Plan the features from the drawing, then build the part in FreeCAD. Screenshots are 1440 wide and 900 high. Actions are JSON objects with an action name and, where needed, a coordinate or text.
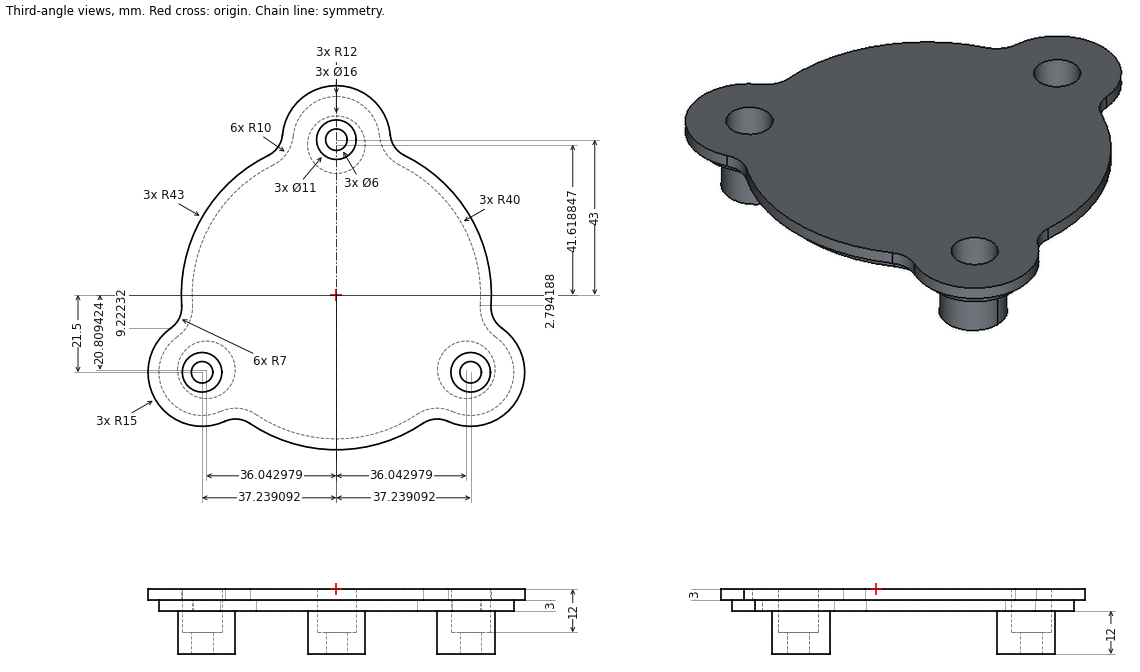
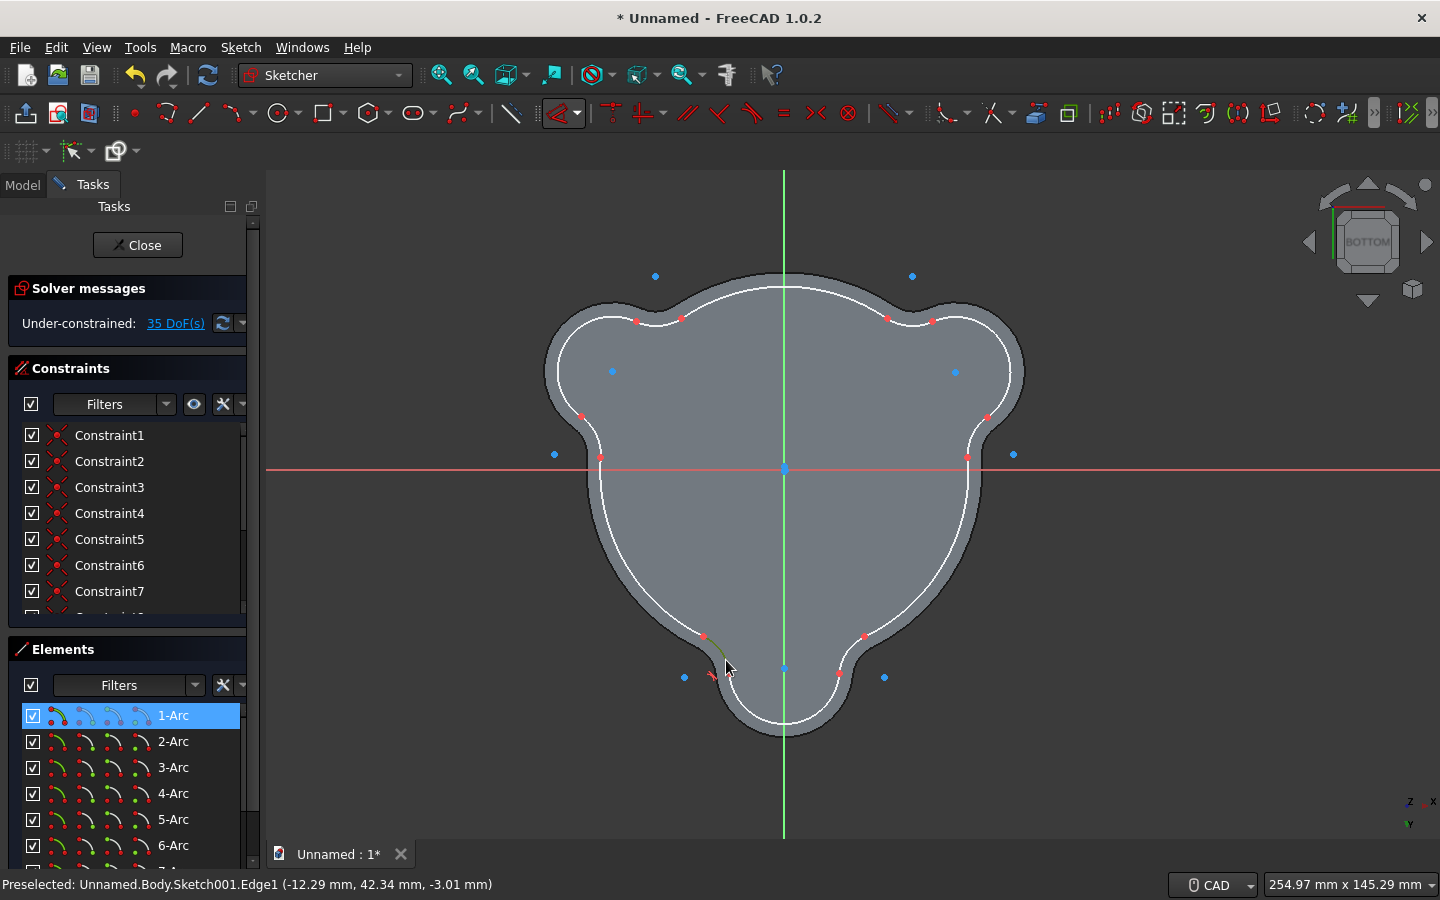
{"action": "left_click", "coordinate": [608, 523]}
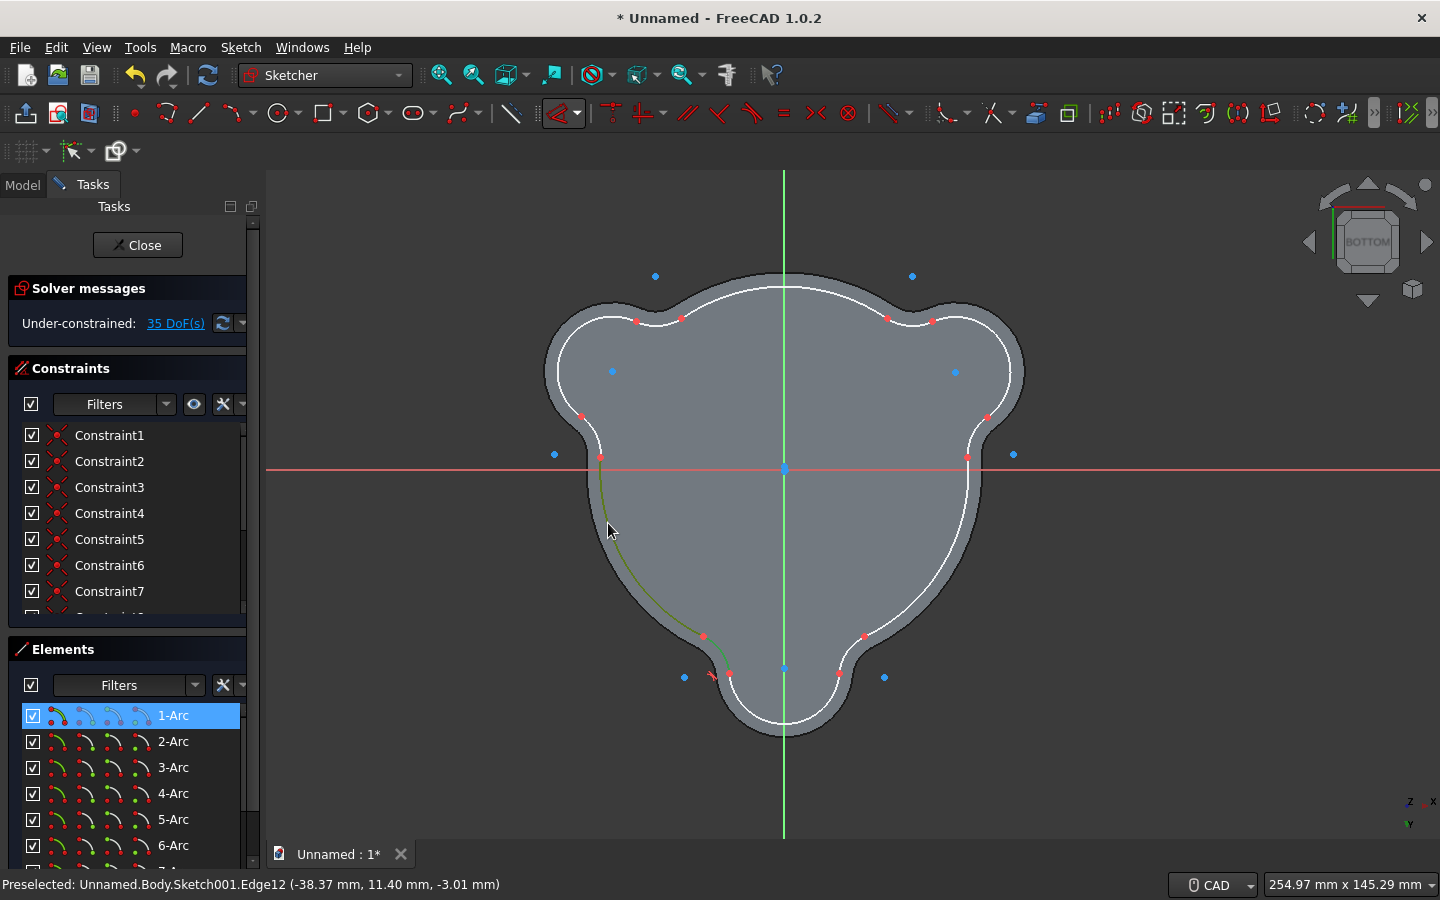
{"action": "left_click", "coordinate": [752, 114]}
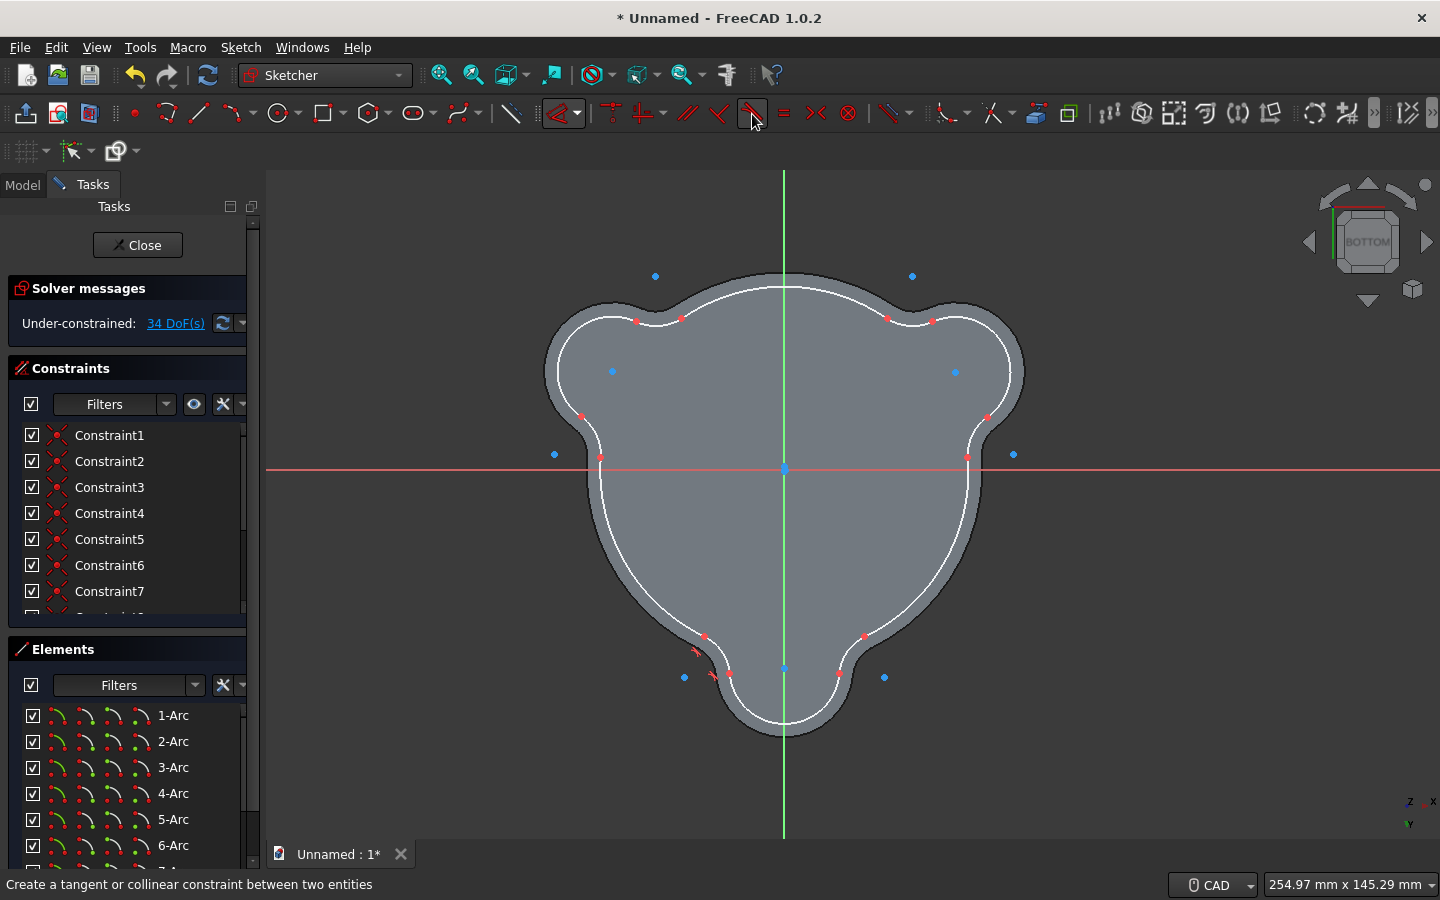
{"action": "left_click", "coordinate": [754, 715]}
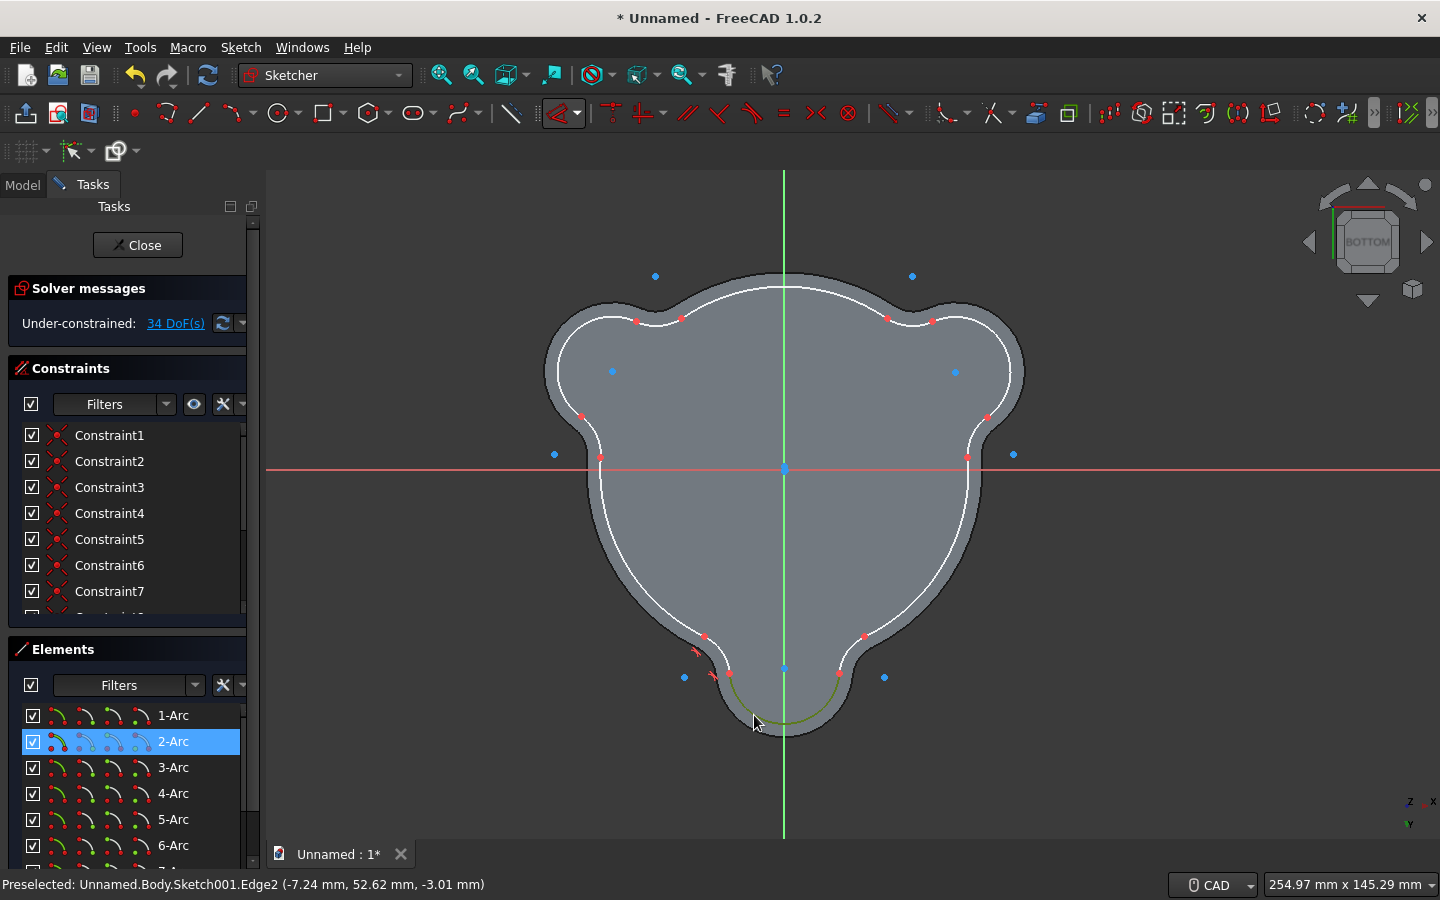
{"action": "left_click", "coordinate": [853, 645]}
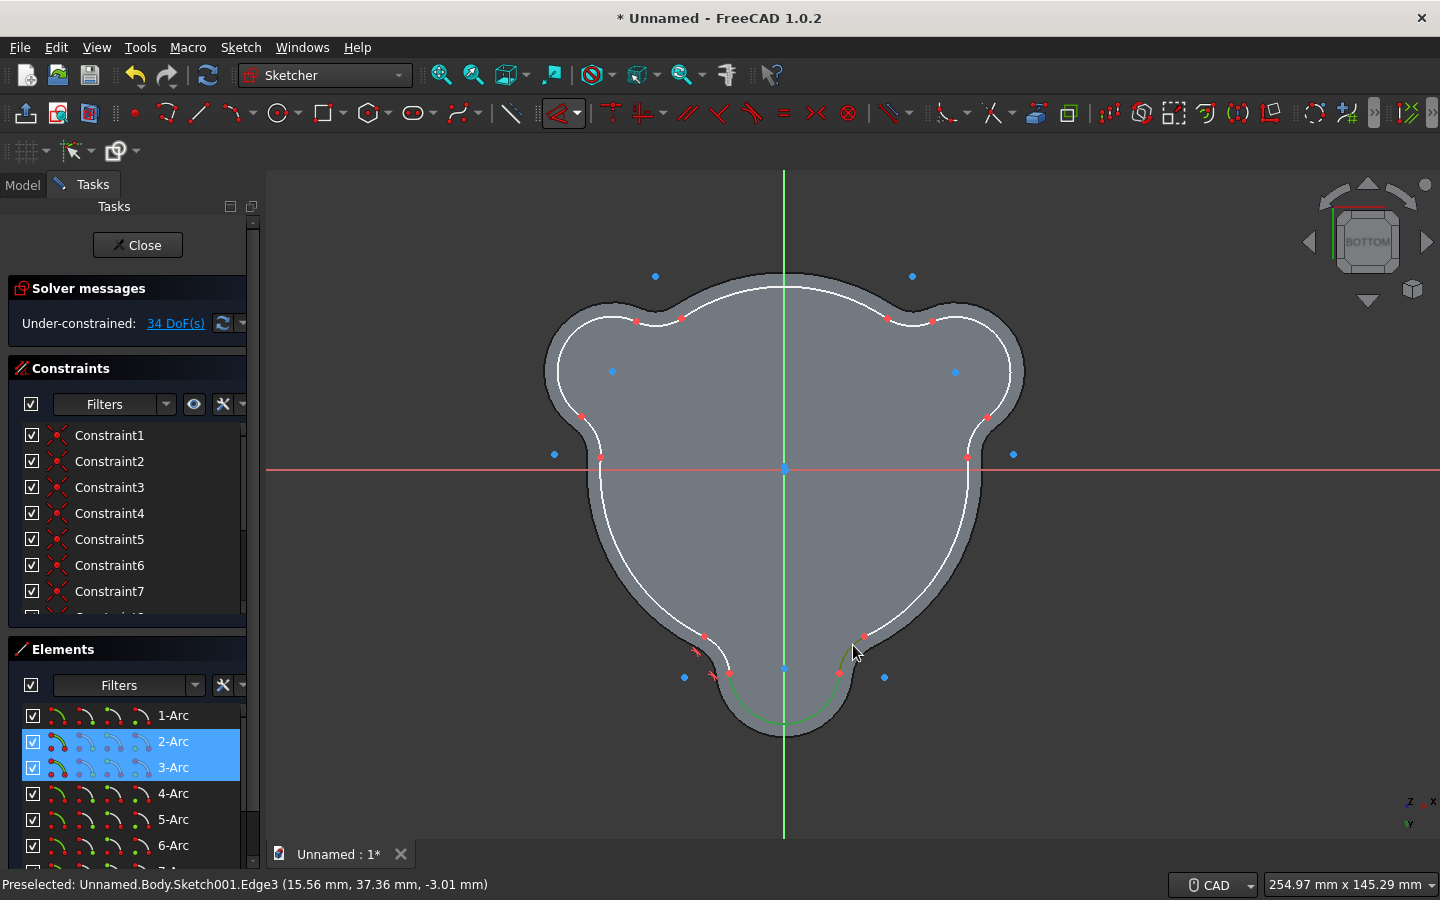
{"action": "left_click", "coordinate": [752, 114]}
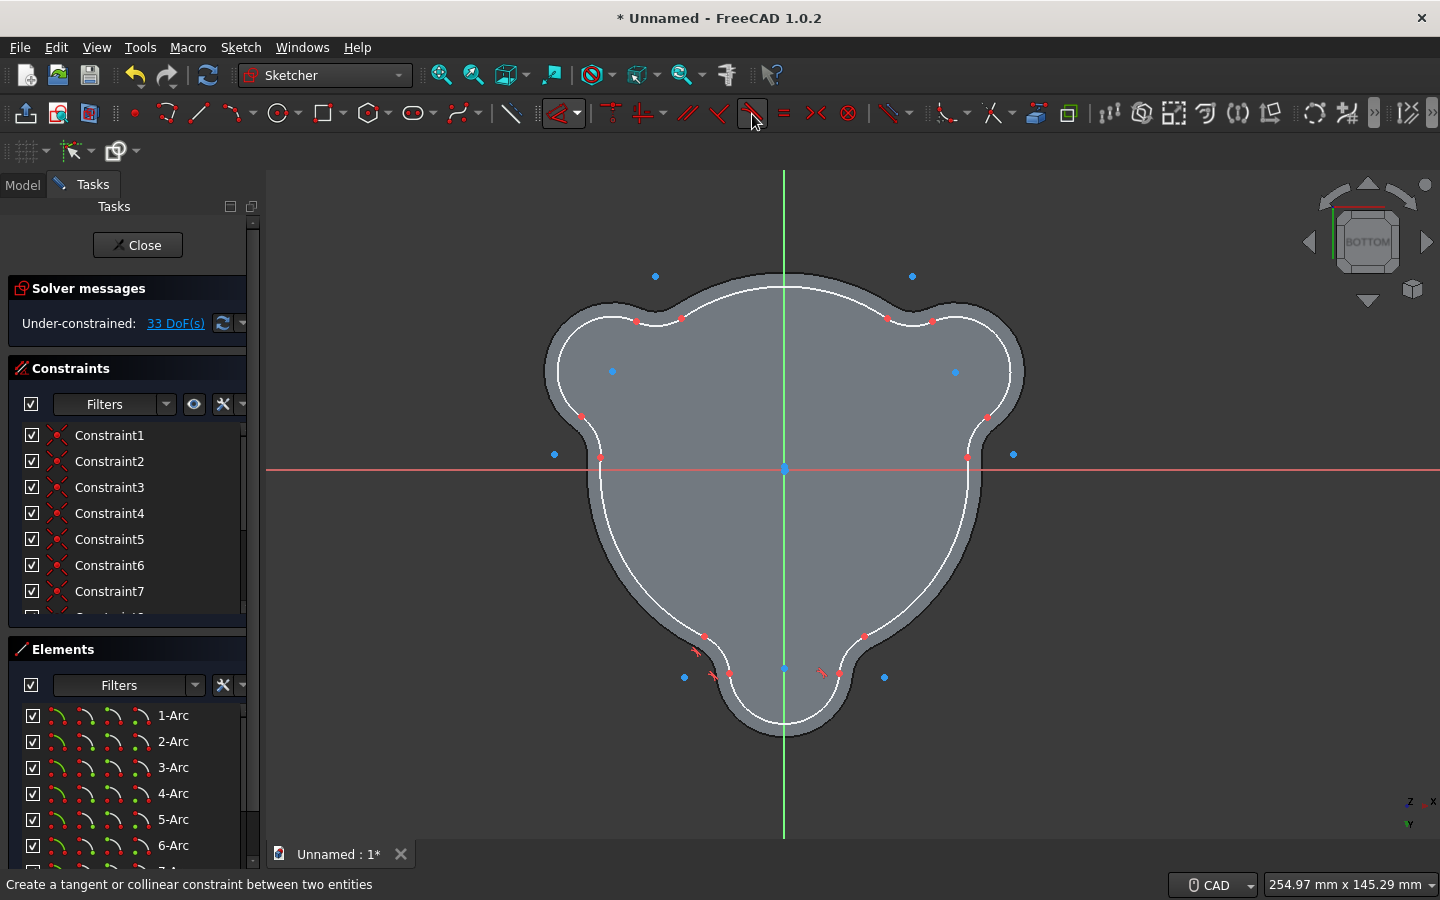
{"action": "left_click", "coordinate": [853, 645]}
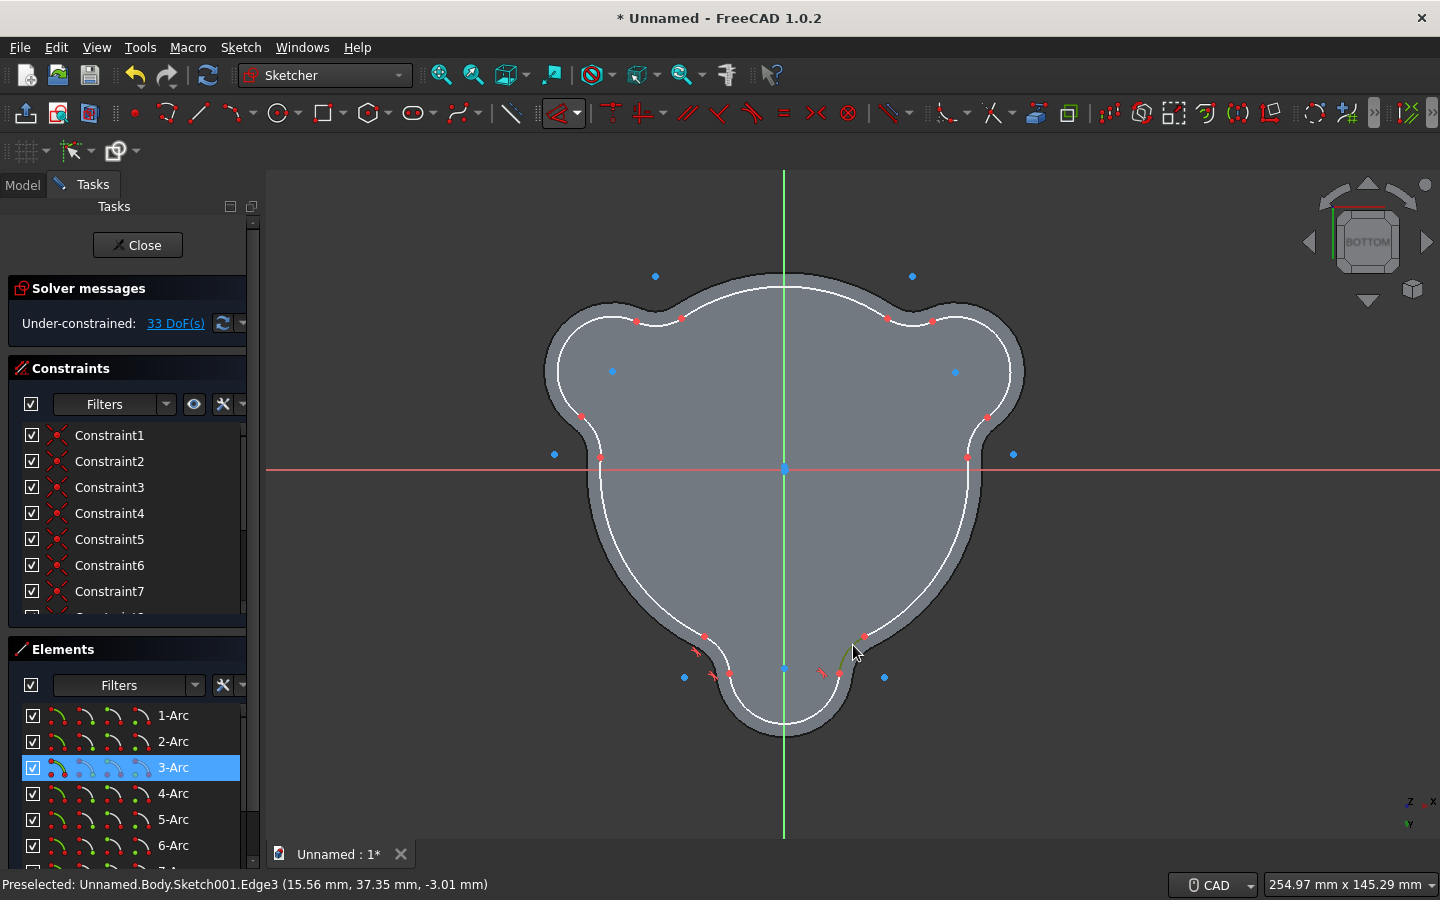
{"action": "left_click", "coordinate": [918, 598]}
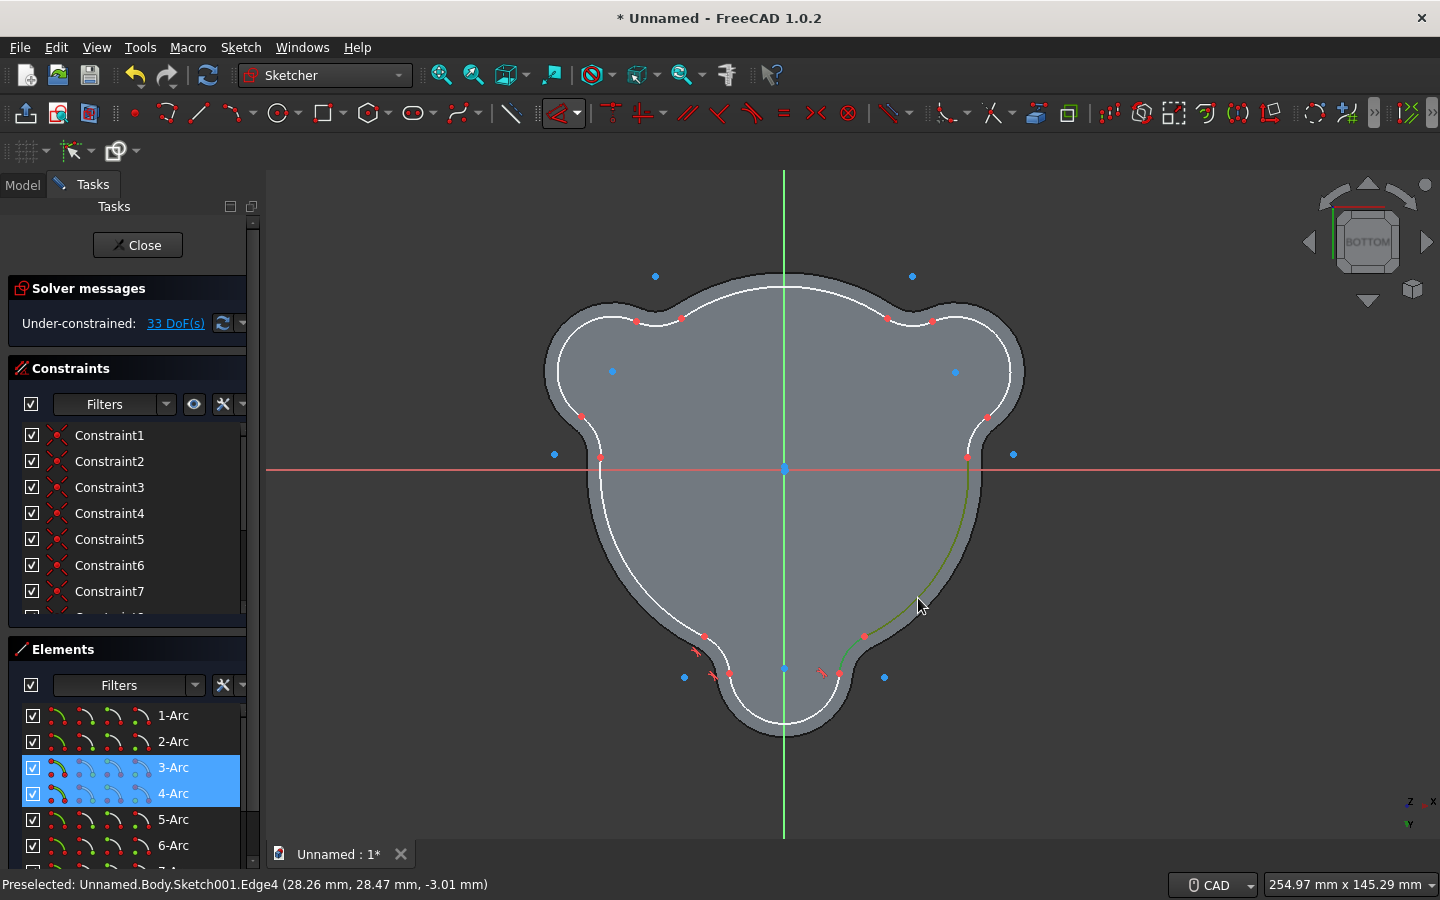
{"action": "left_click", "coordinate": [752, 114]}